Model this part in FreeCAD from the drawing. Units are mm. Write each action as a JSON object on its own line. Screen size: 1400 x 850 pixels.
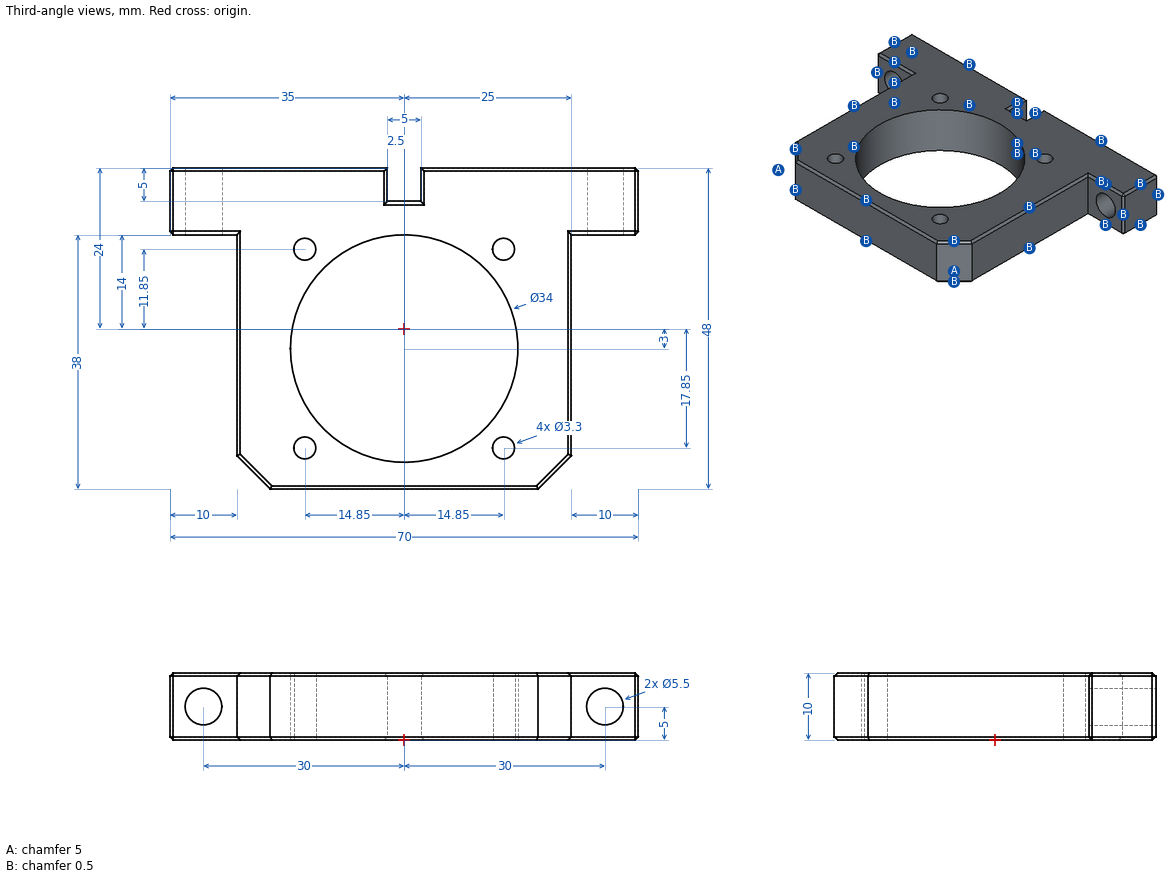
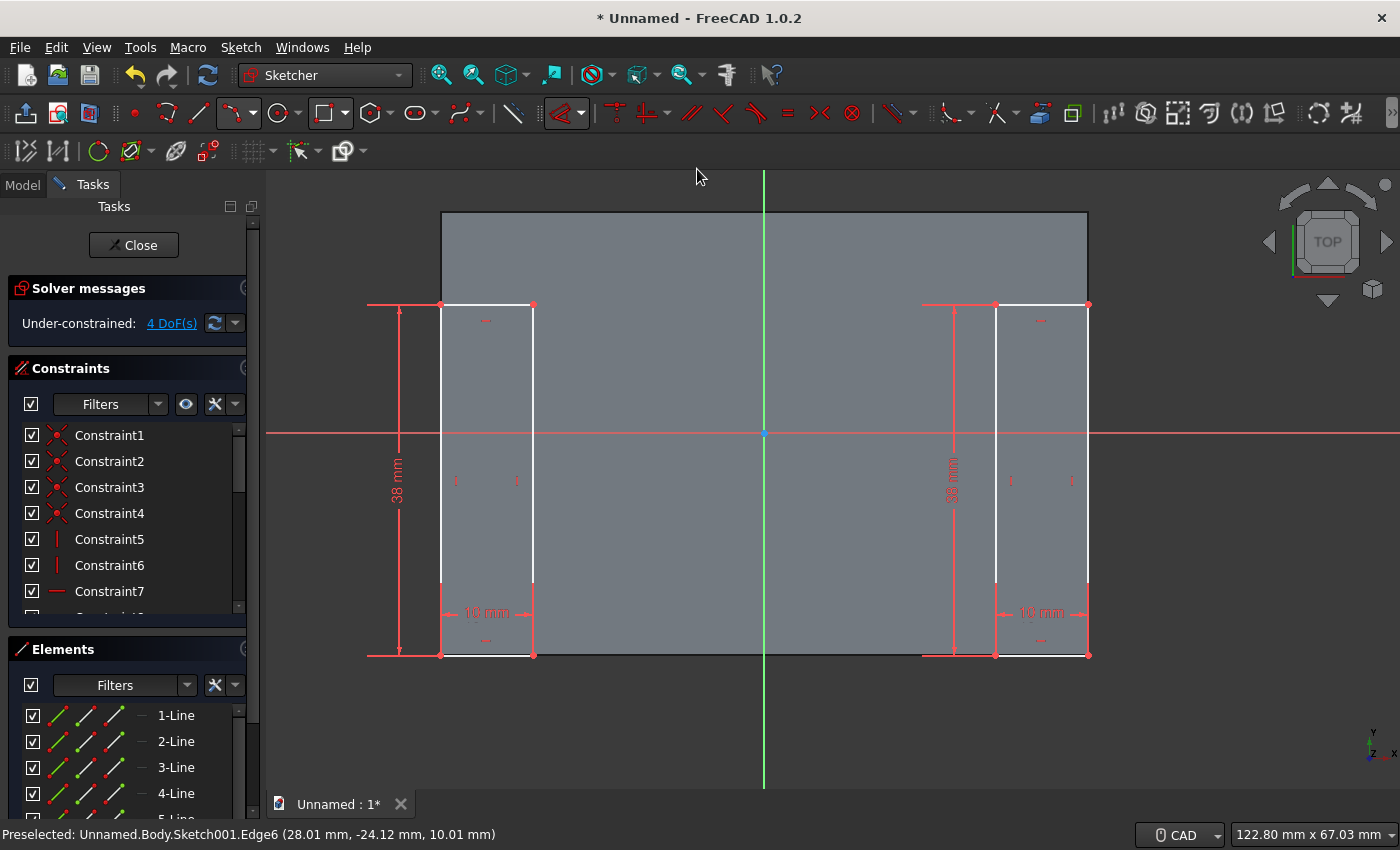
{"action": "left_click", "coordinate": [441, 305]}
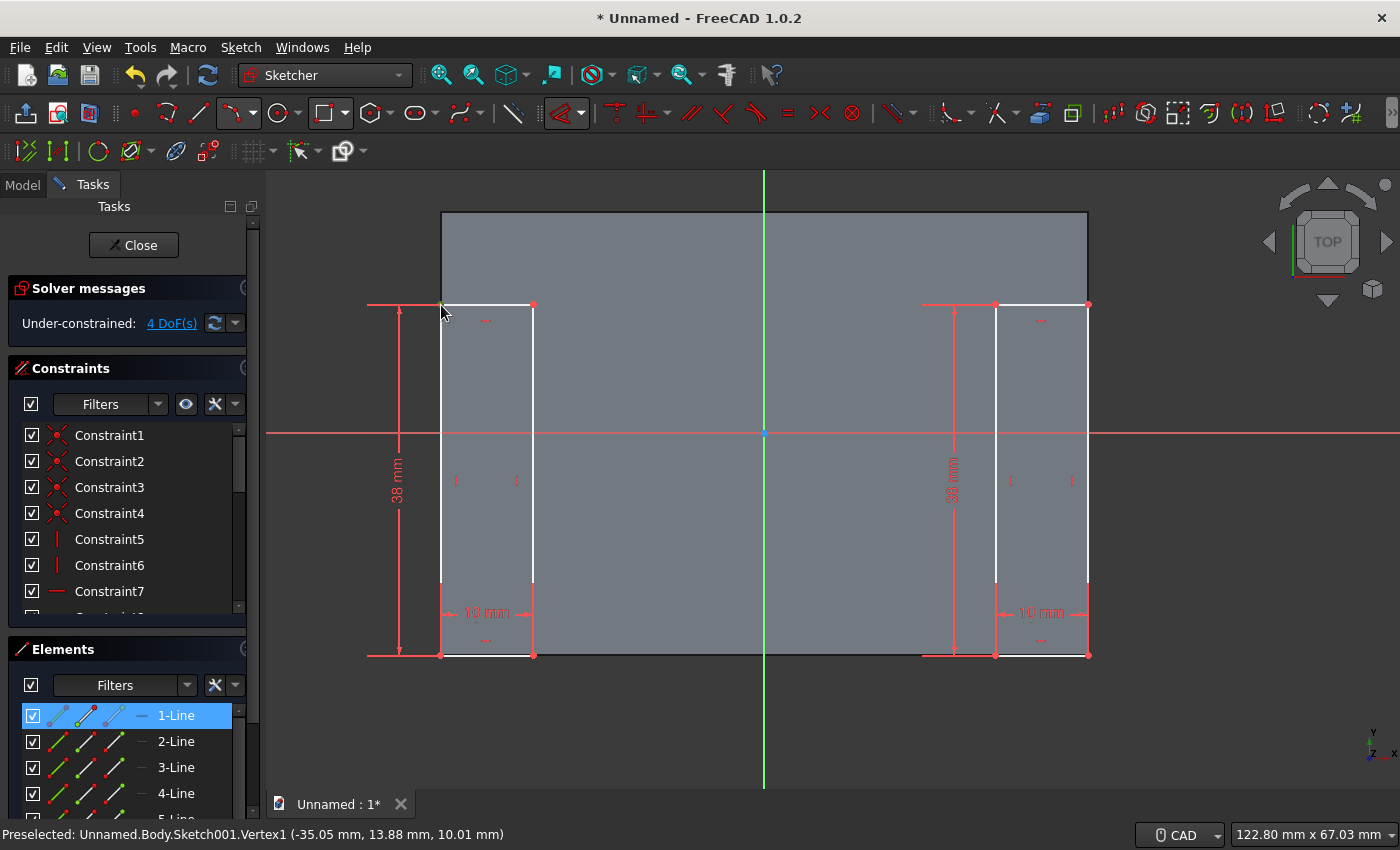
{"action": "key", "text": "l"}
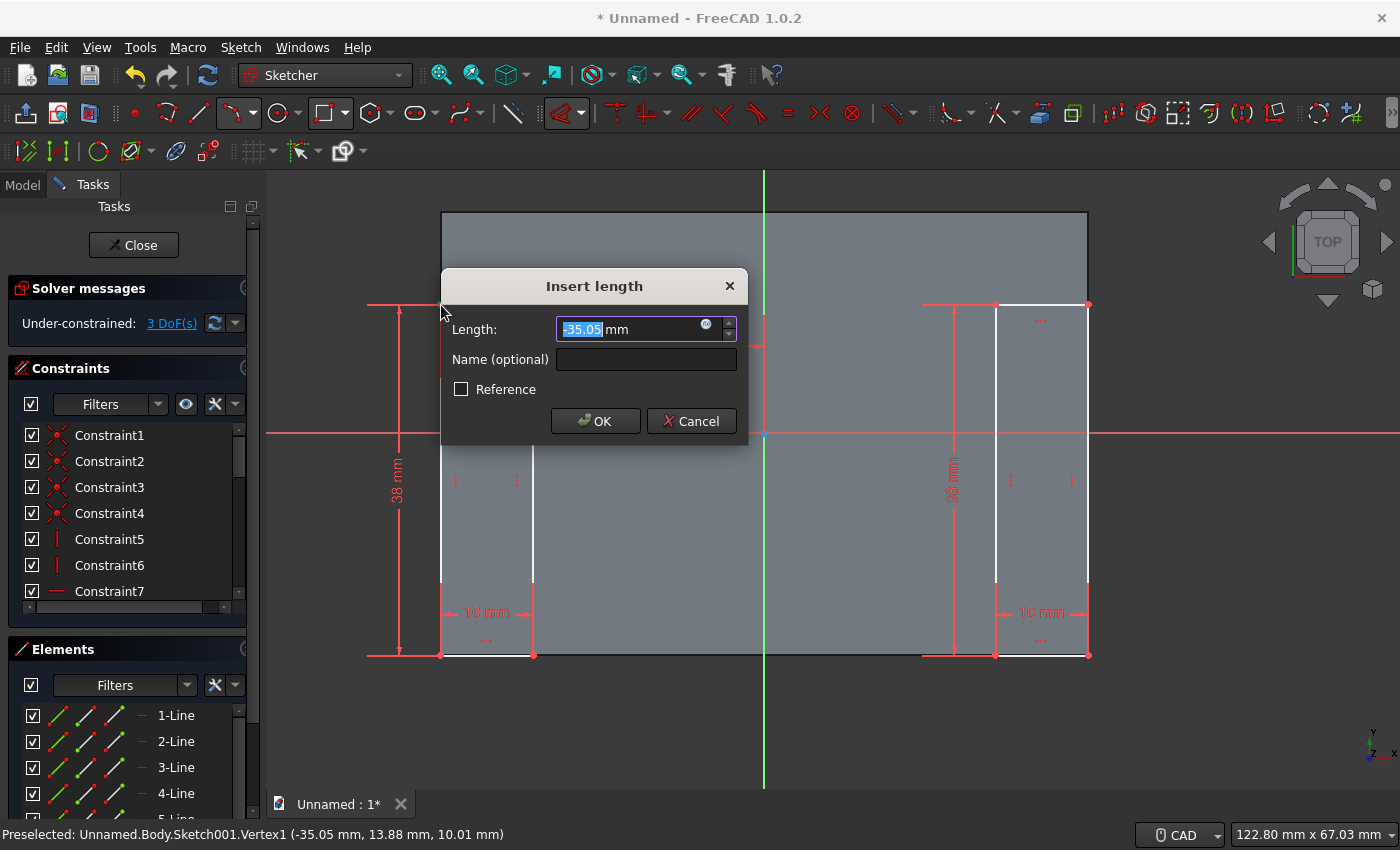
{"action": "type", "text": "-35"}
{"action": "key", "text": "Return"}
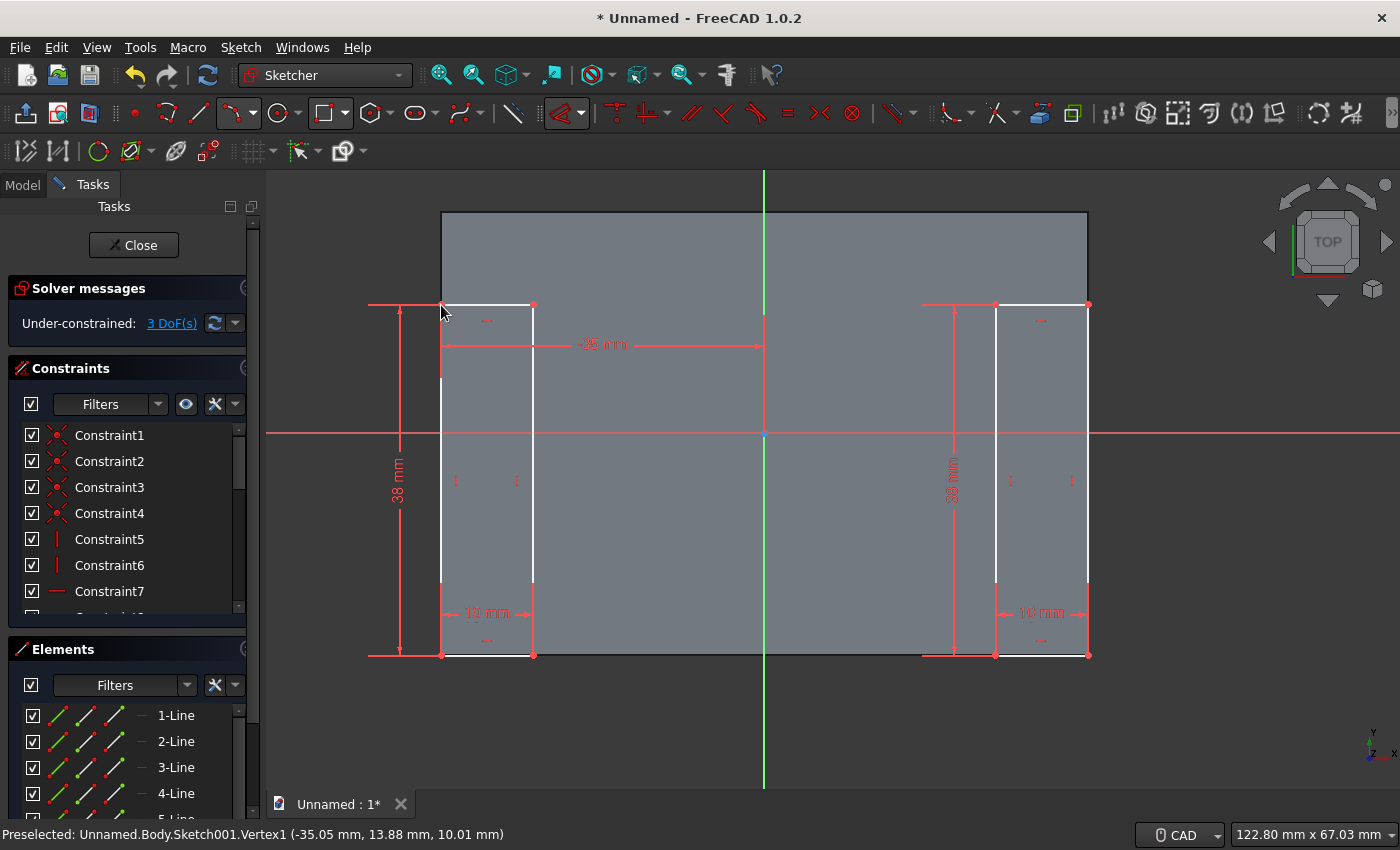
{"action": "left_click", "coordinate": [441, 305]}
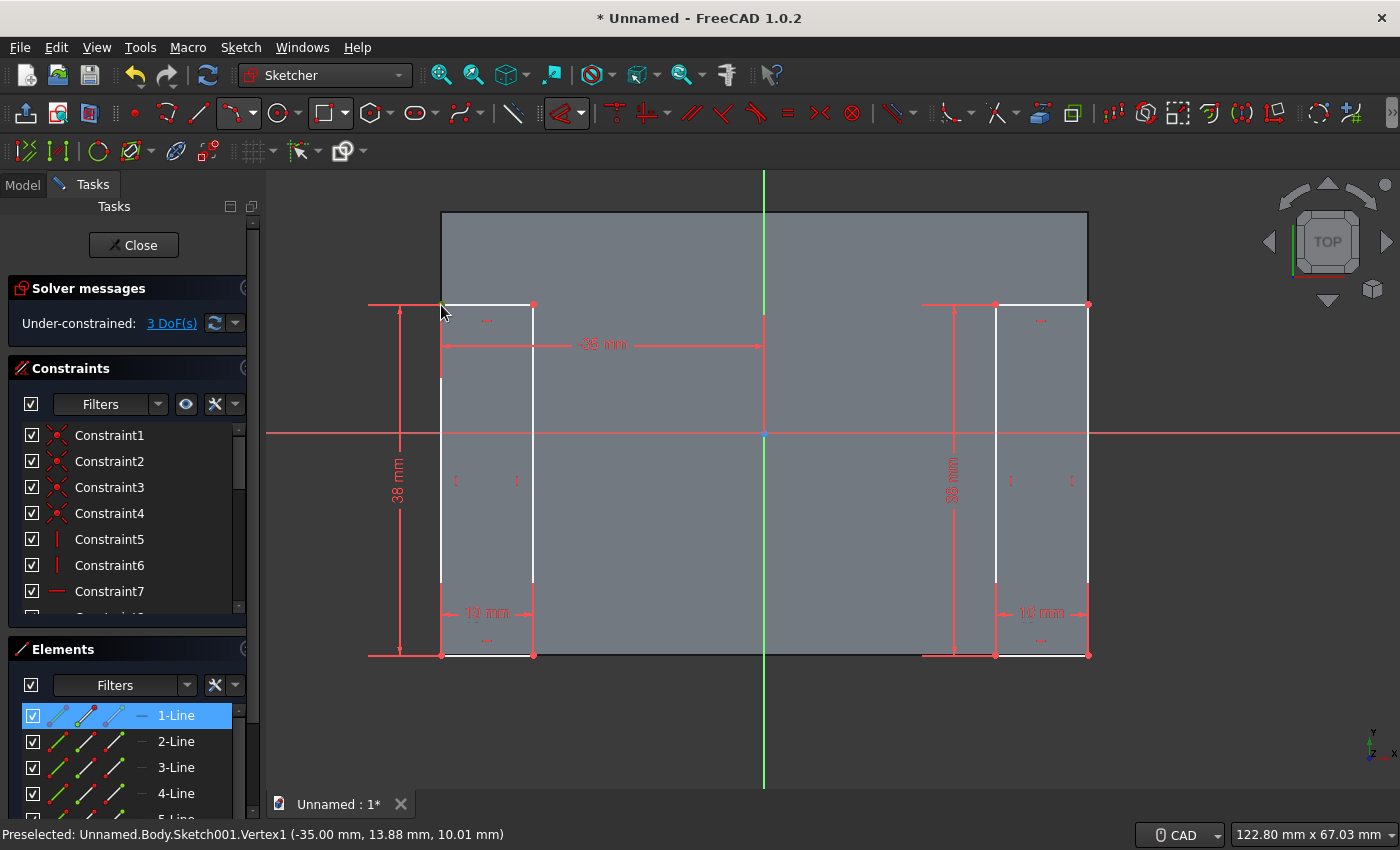
{"action": "key", "text": "i"}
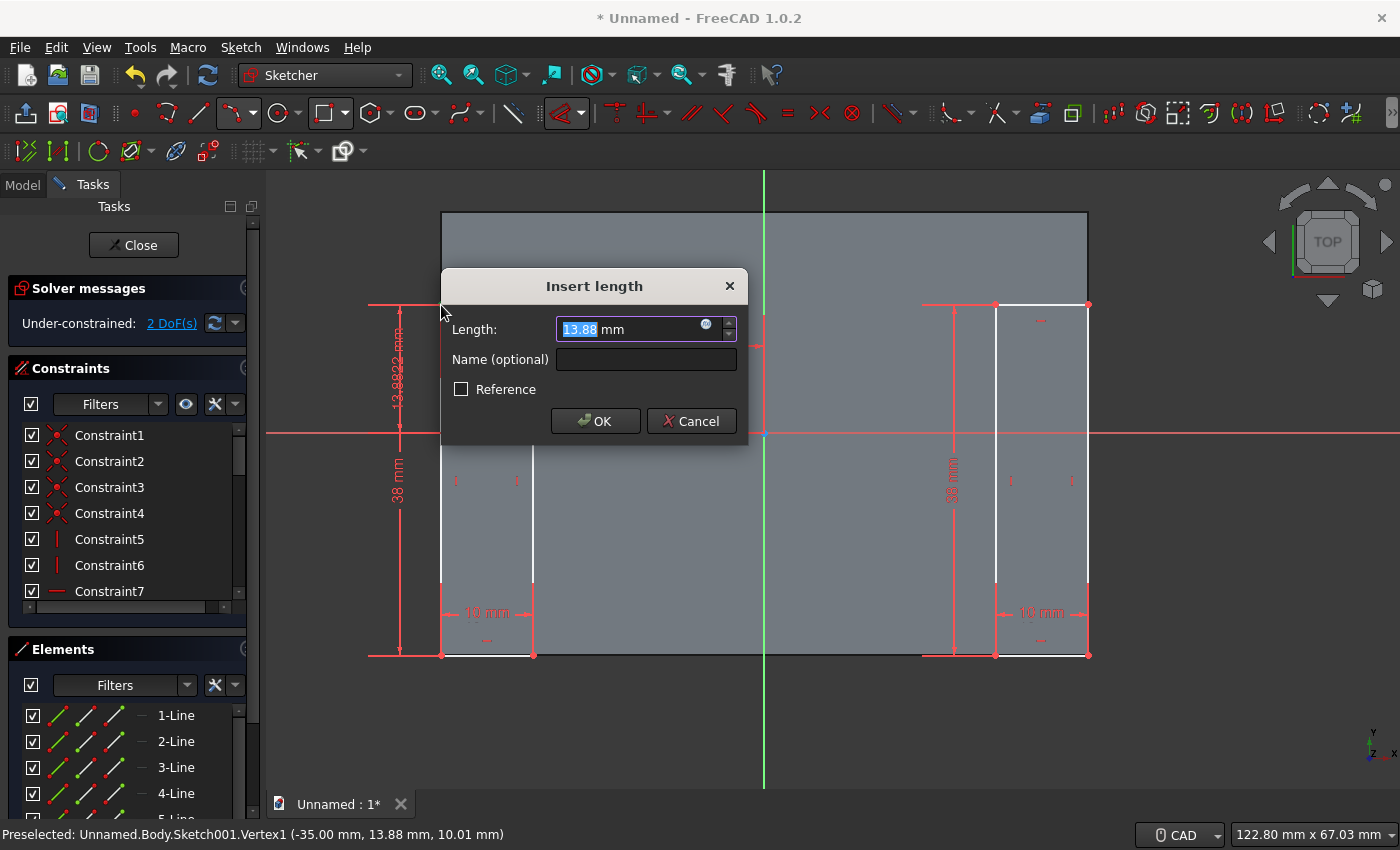
{"action": "type", "text": "14"}
{"action": "key", "text": "Return"}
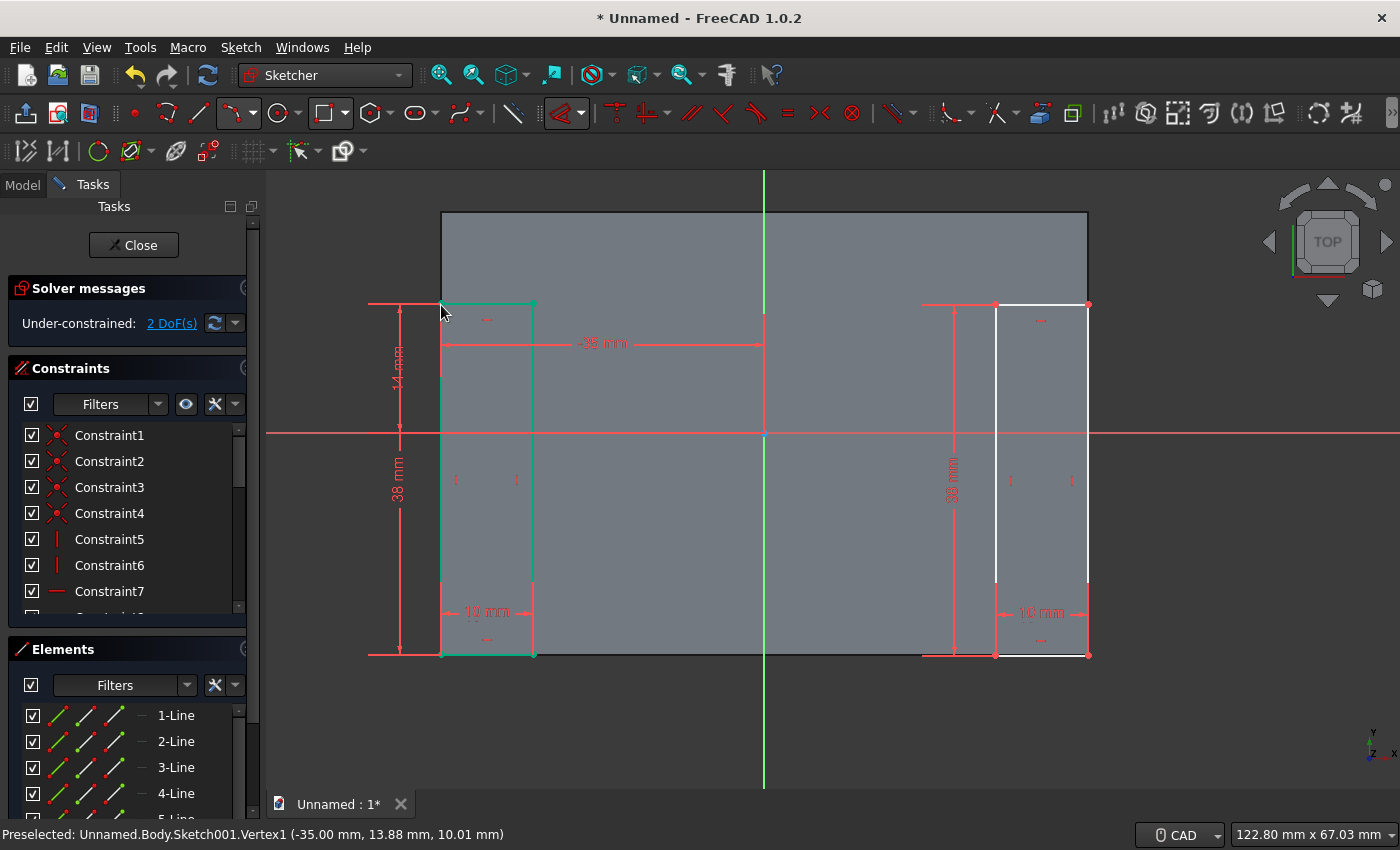
{"action": "left_click", "coordinate": [996, 305]}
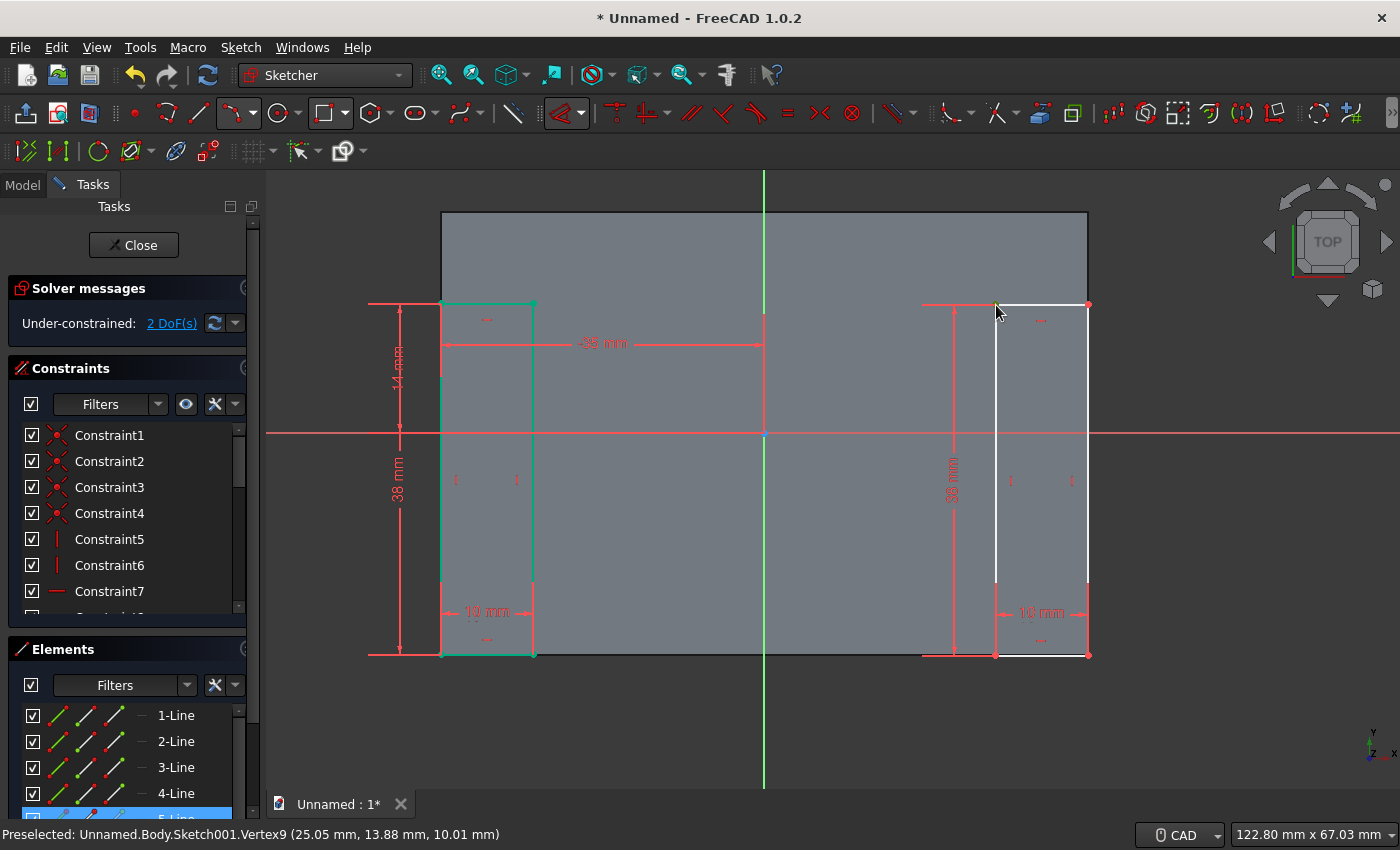
{"action": "left_click", "coordinate": [584, 114]}